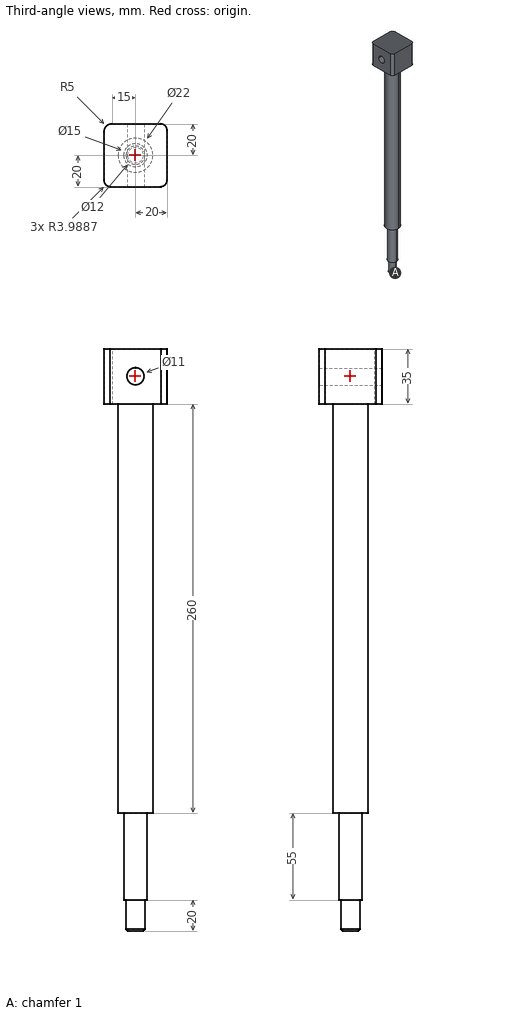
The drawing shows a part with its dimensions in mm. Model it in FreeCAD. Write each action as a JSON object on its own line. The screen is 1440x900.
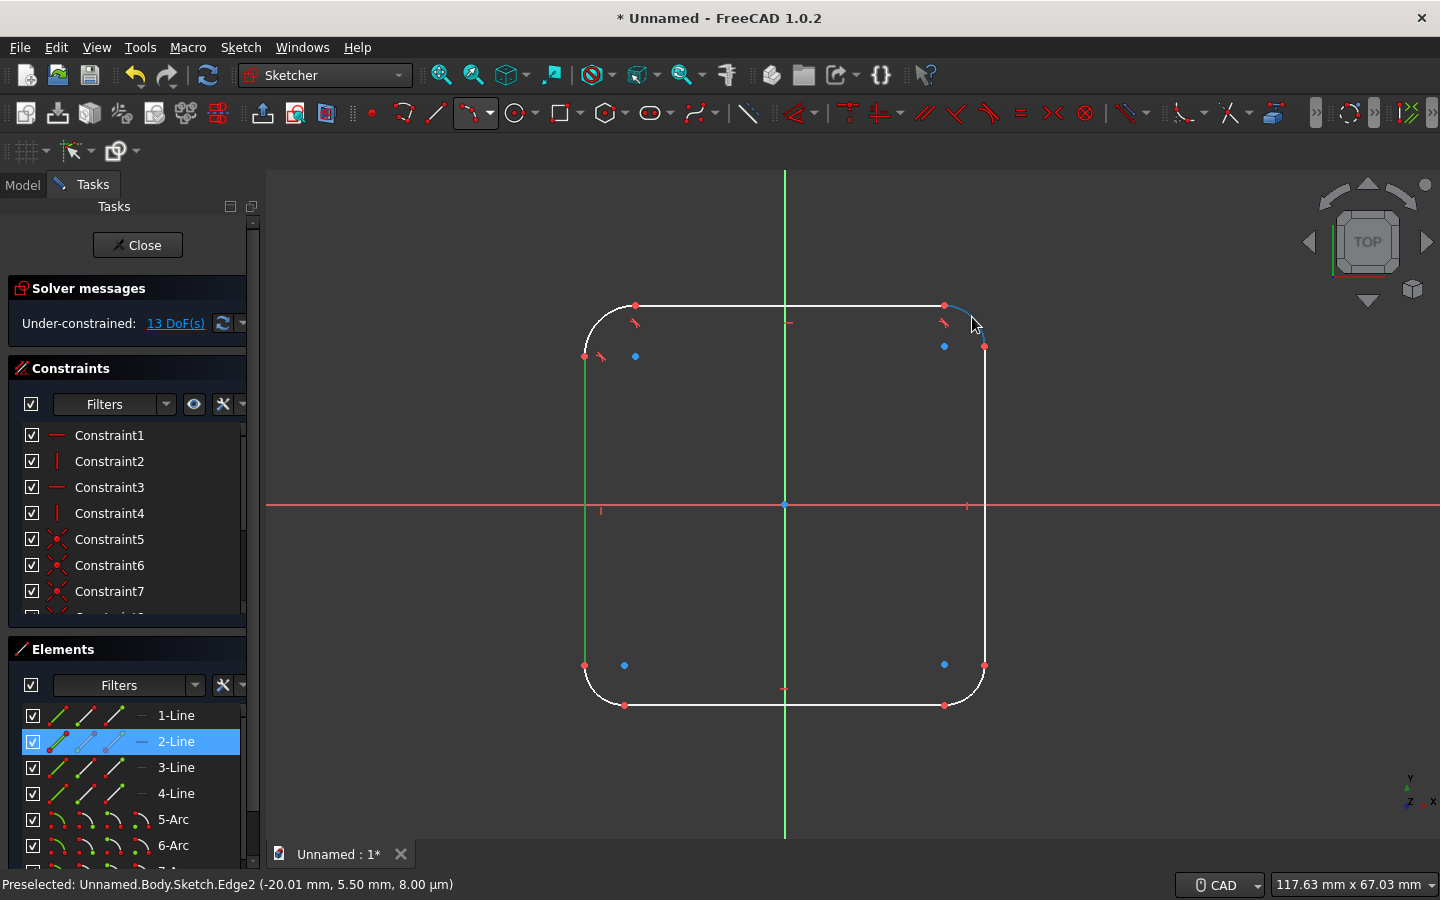
{"action": "left_click", "coordinate": [589, 683]}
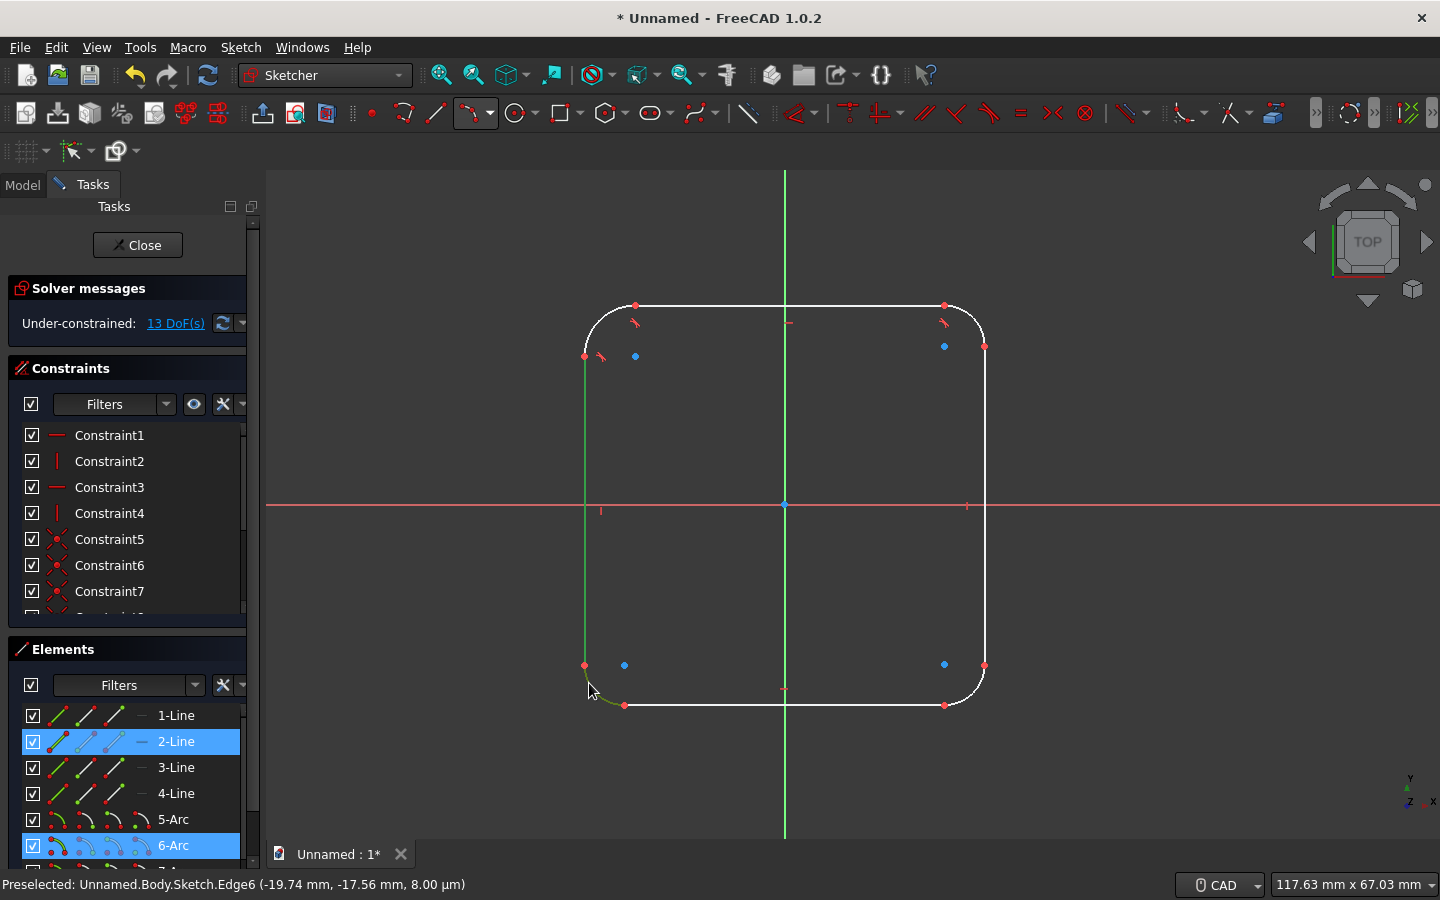
{"action": "left_click", "coordinate": [990, 114]}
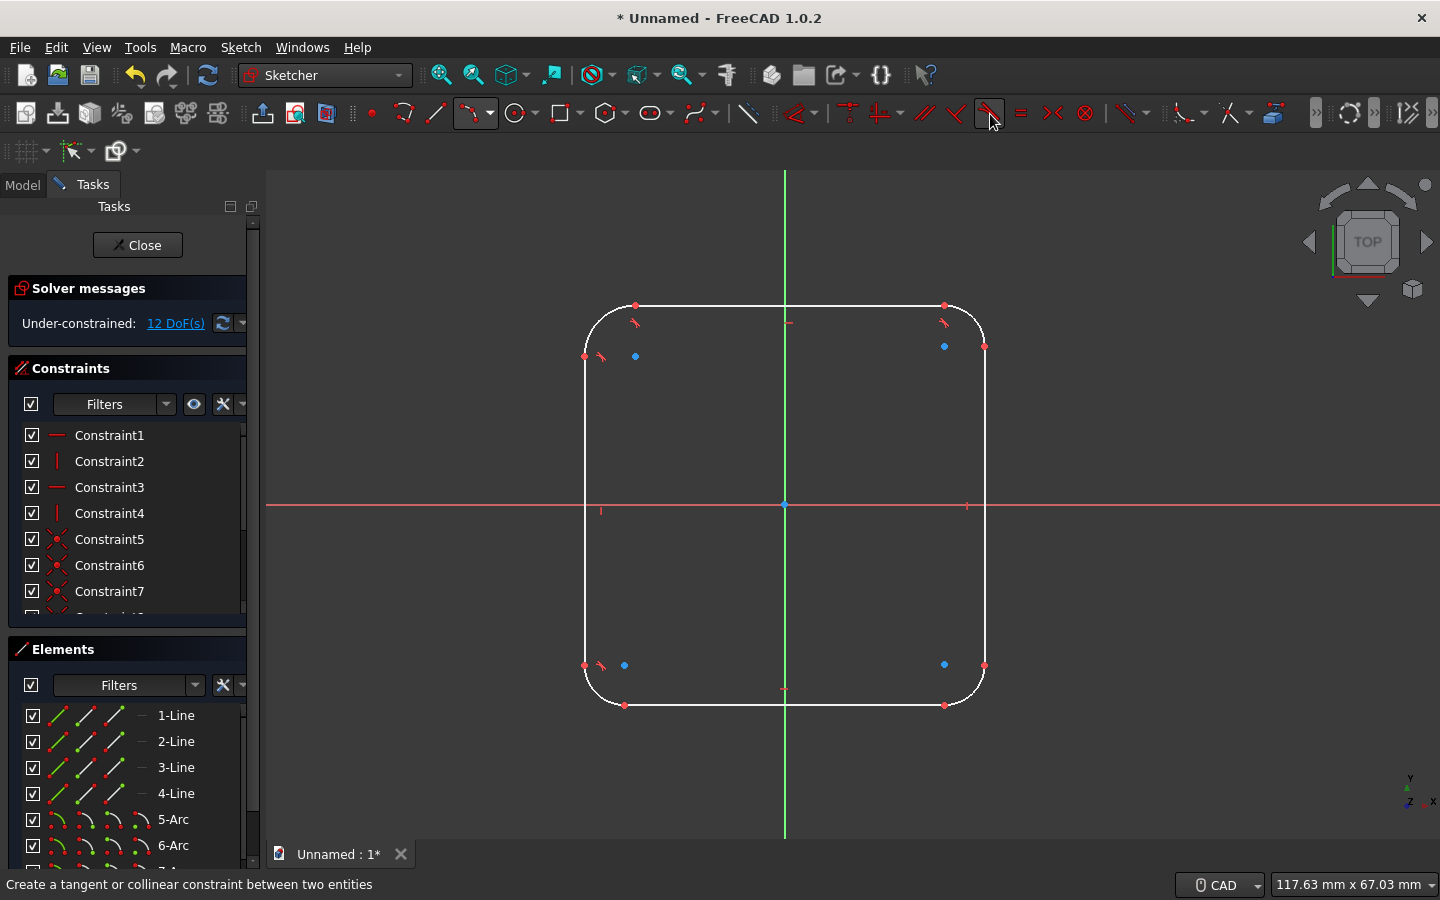
{"action": "left_click", "coordinate": [721, 705]}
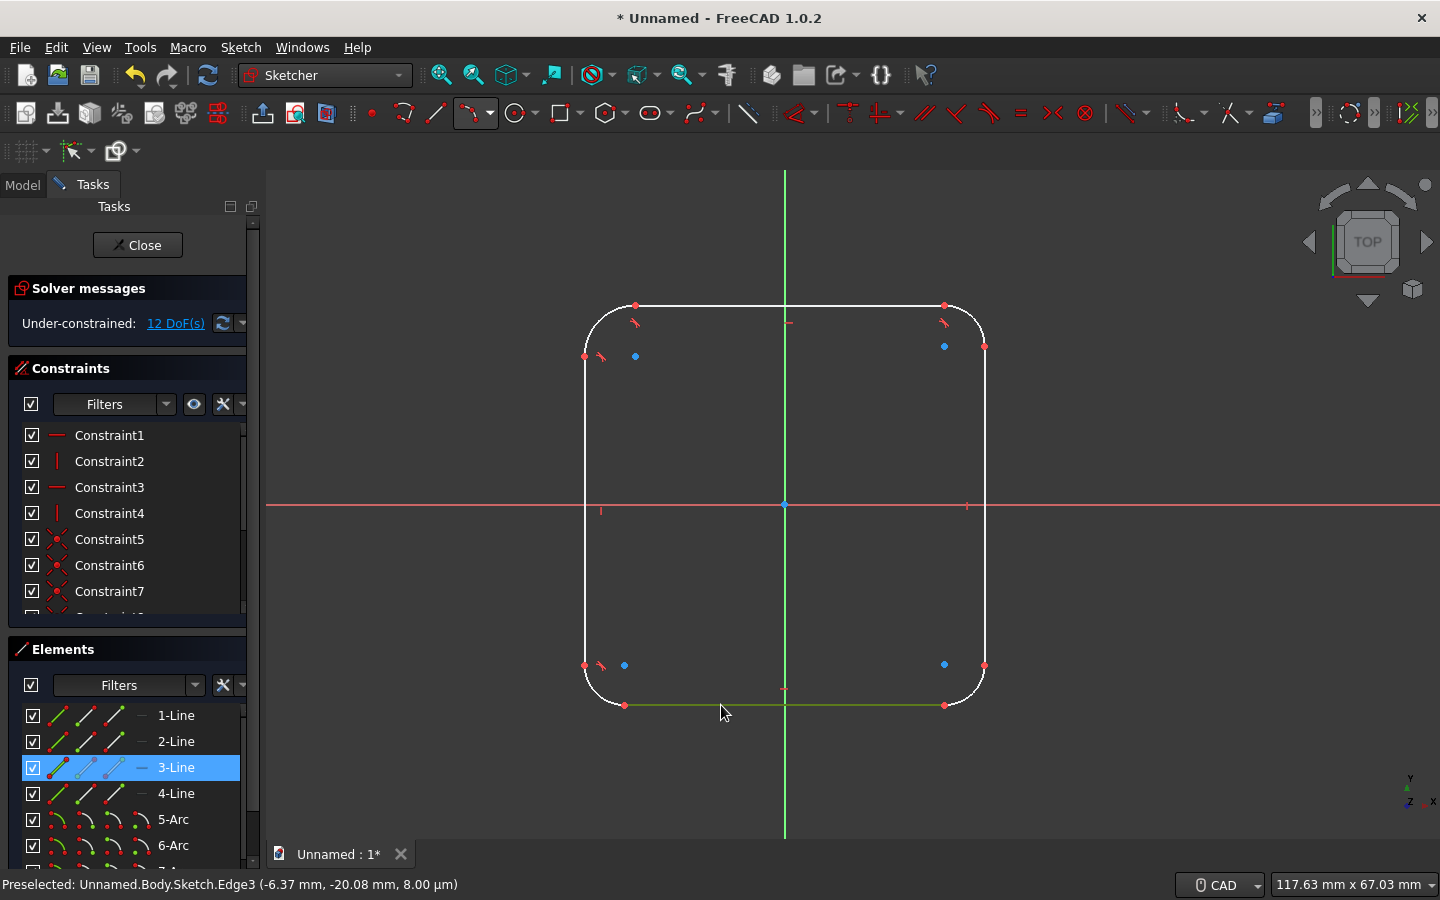
{"action": "left_click", "coordinate": [589, 683]}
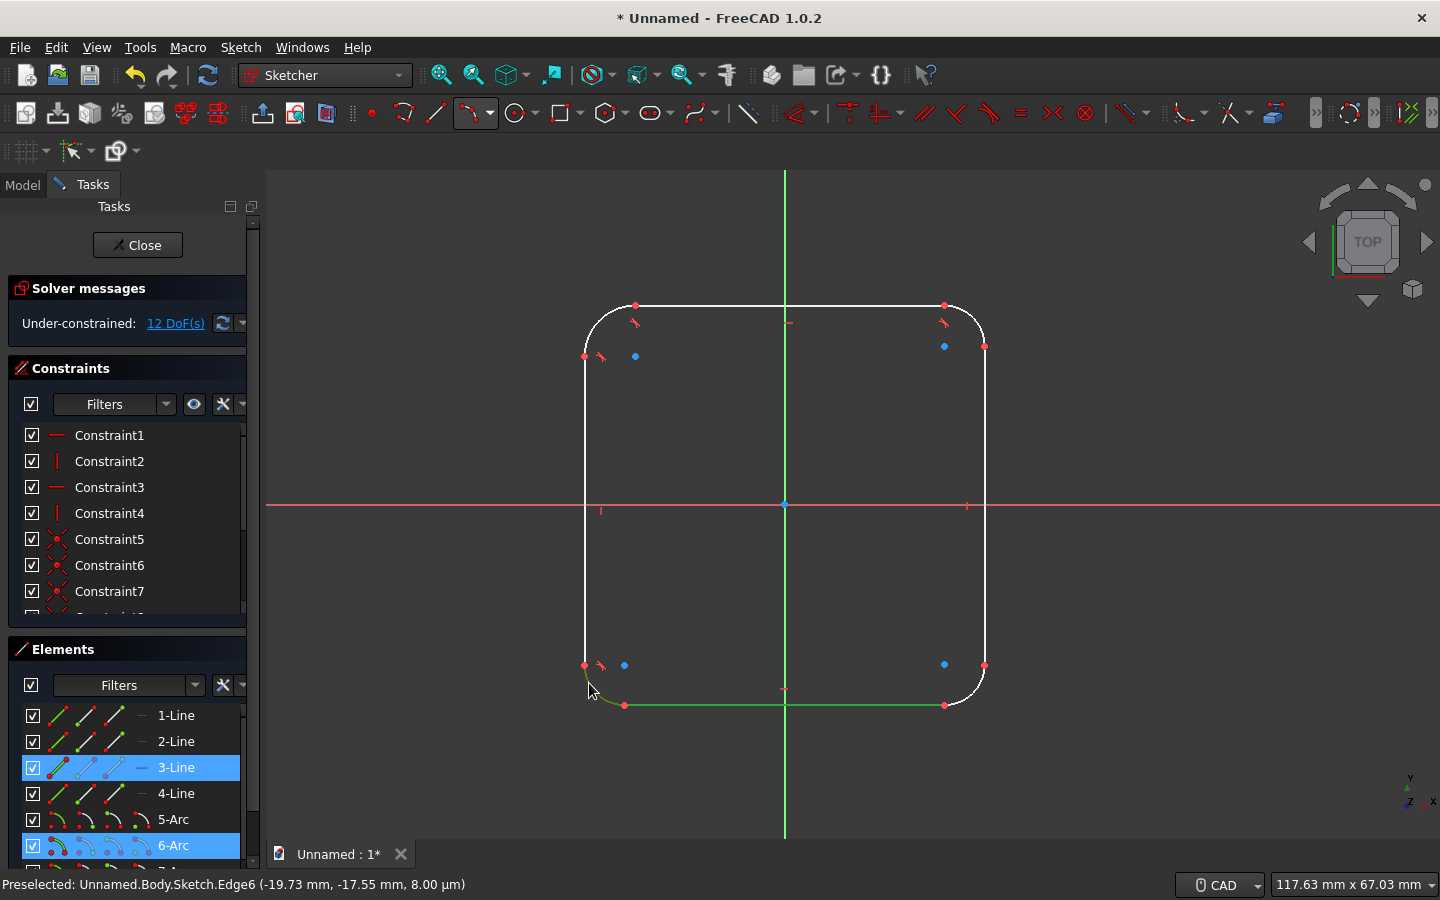
{"action": "key", "text": "t"}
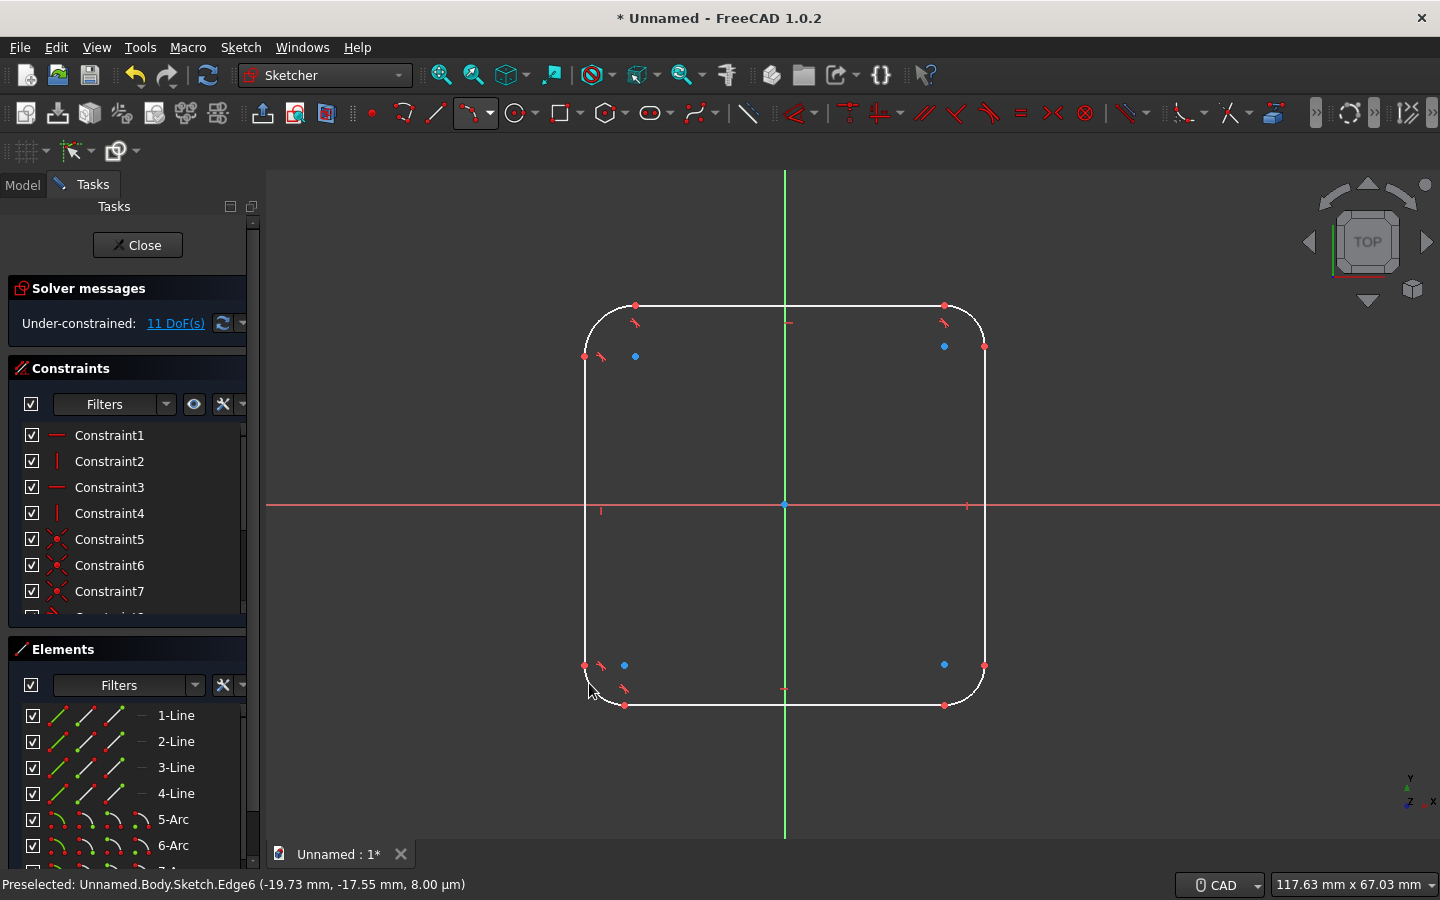
{"action": "left_click", "coordinate": [721, 705]}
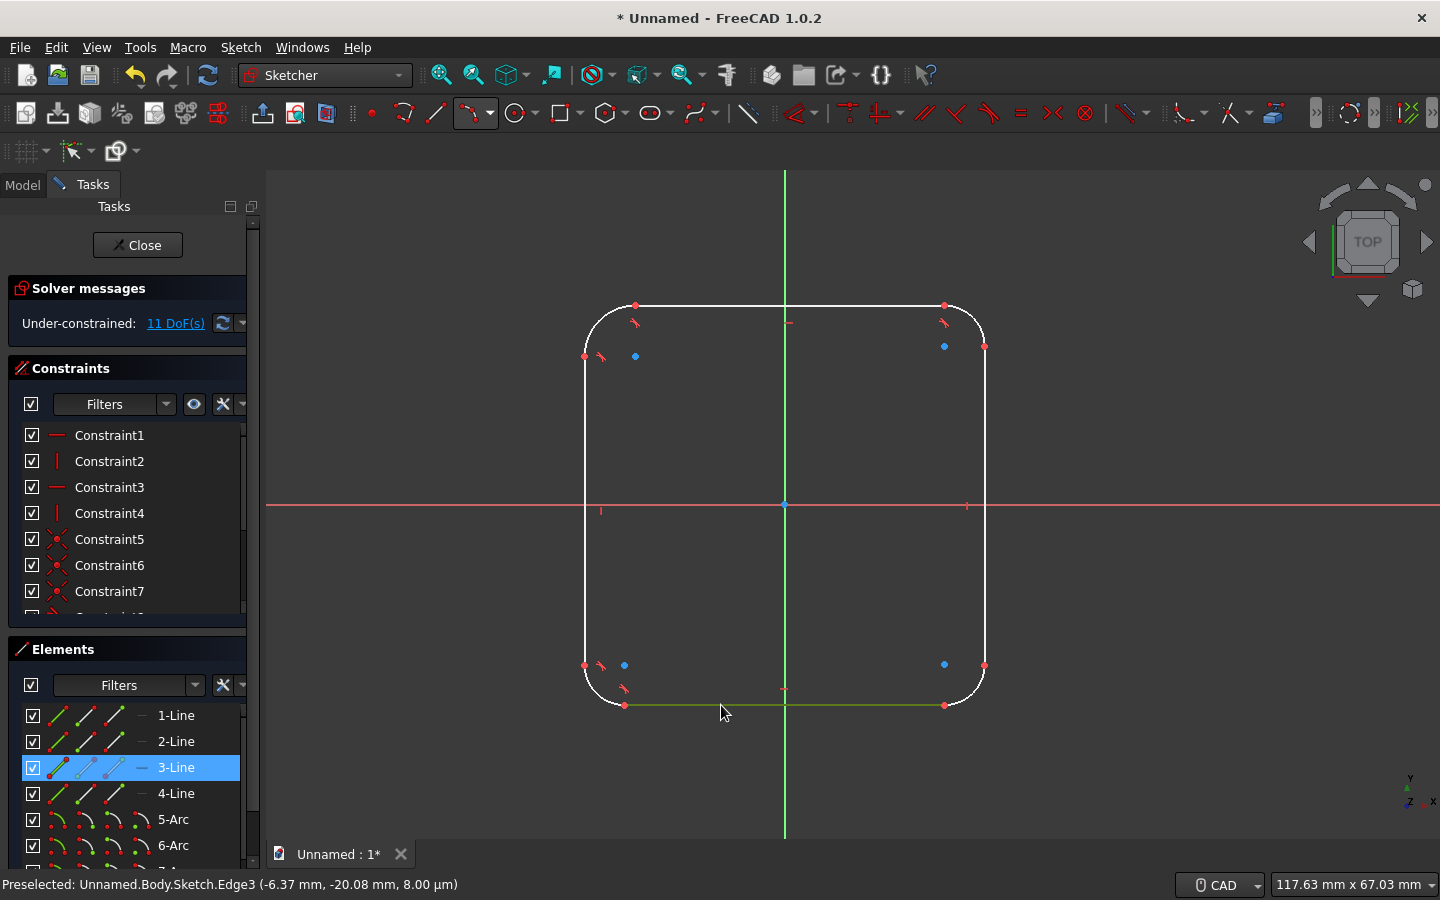
{"action": "left_click", "coordinate": [963, 701]}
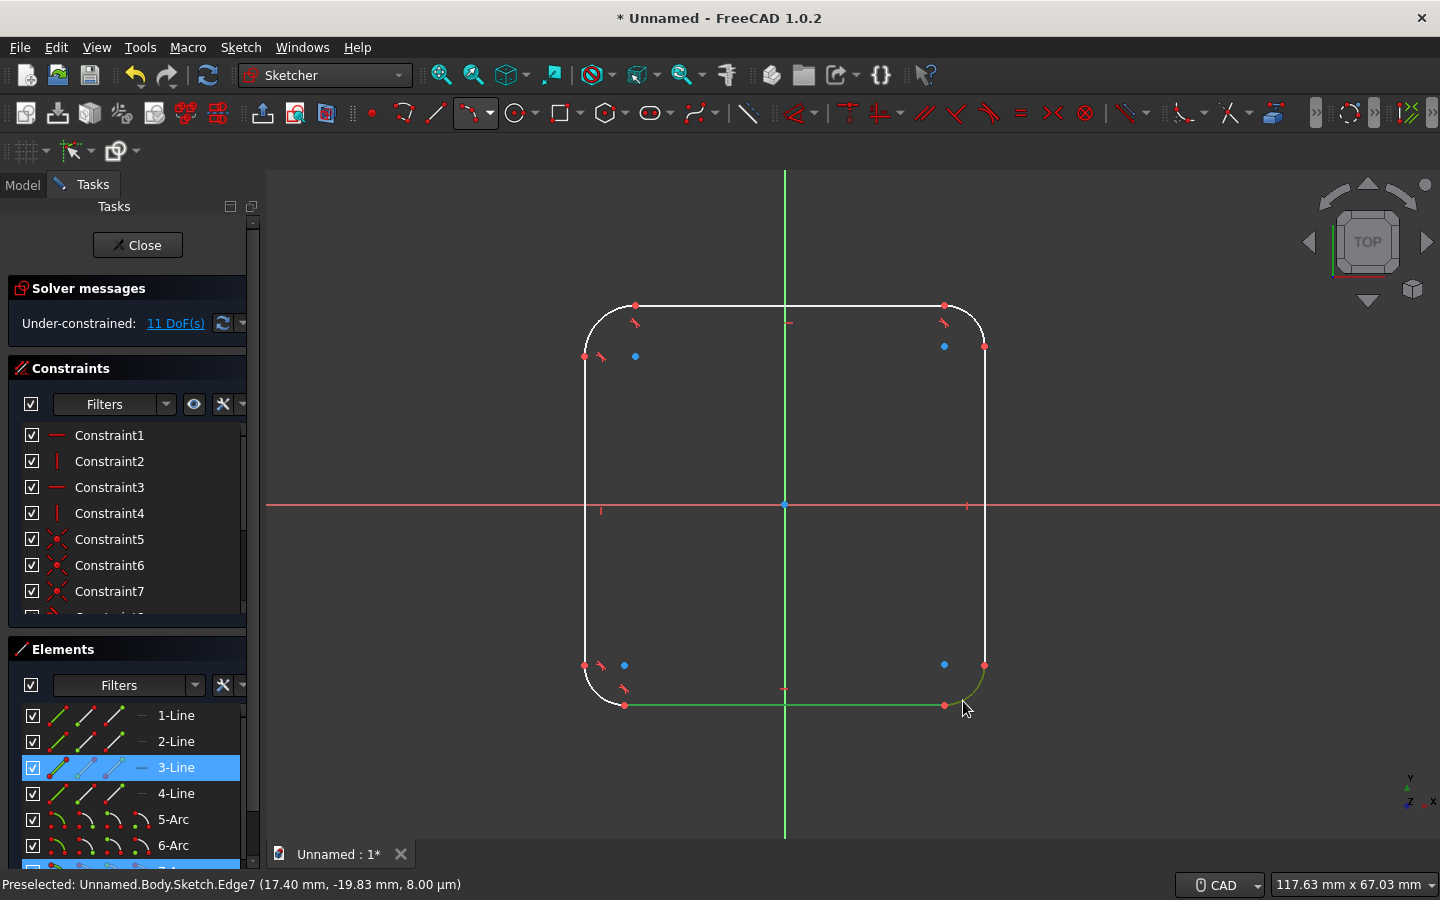
{"action": "left_click", "coordinate": [990, 114]}